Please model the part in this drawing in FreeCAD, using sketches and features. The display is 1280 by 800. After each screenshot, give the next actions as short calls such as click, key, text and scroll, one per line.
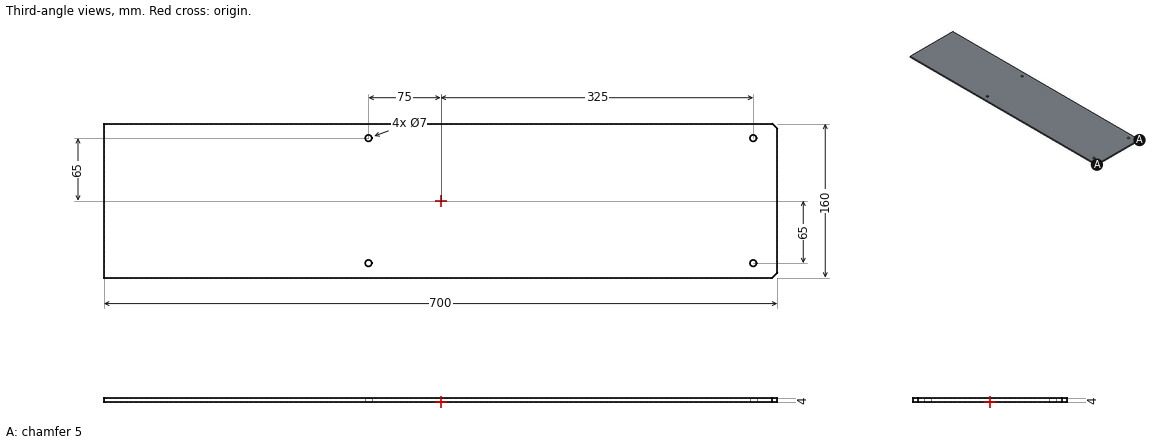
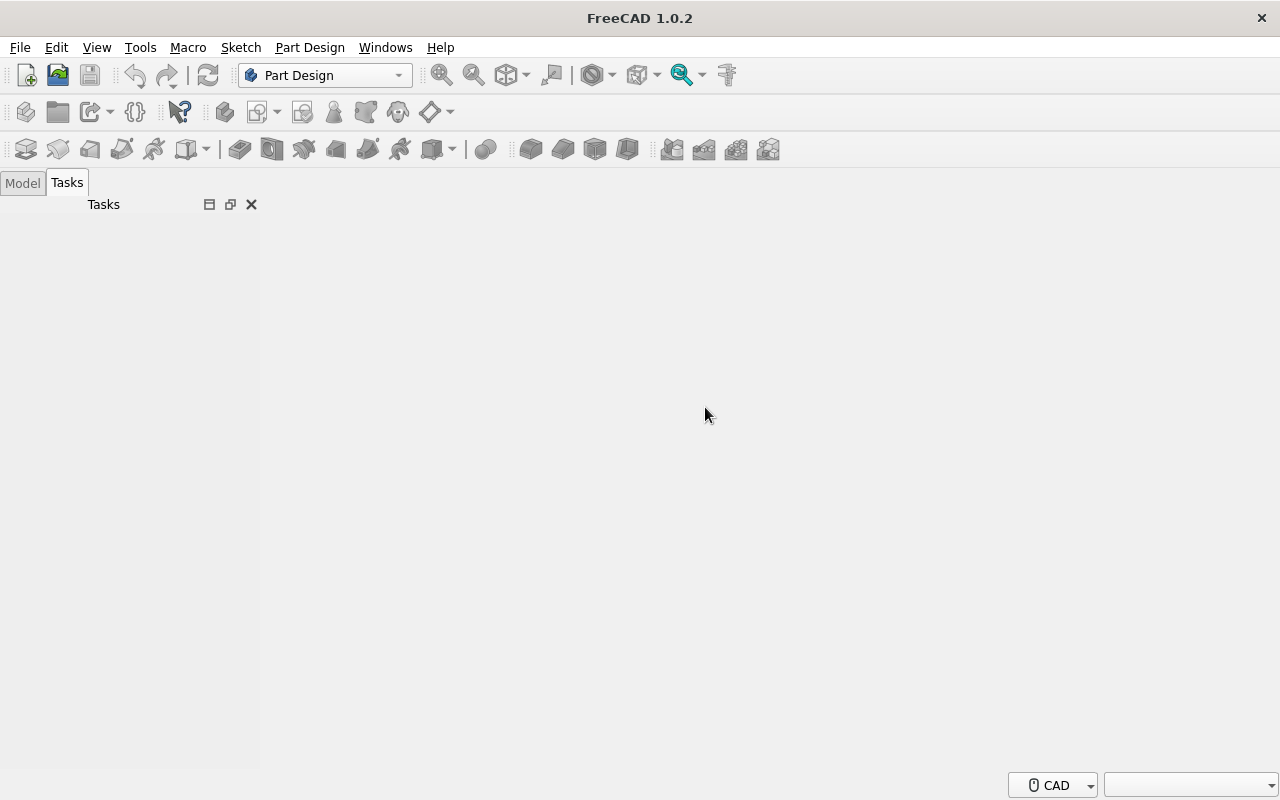
click(26, 76)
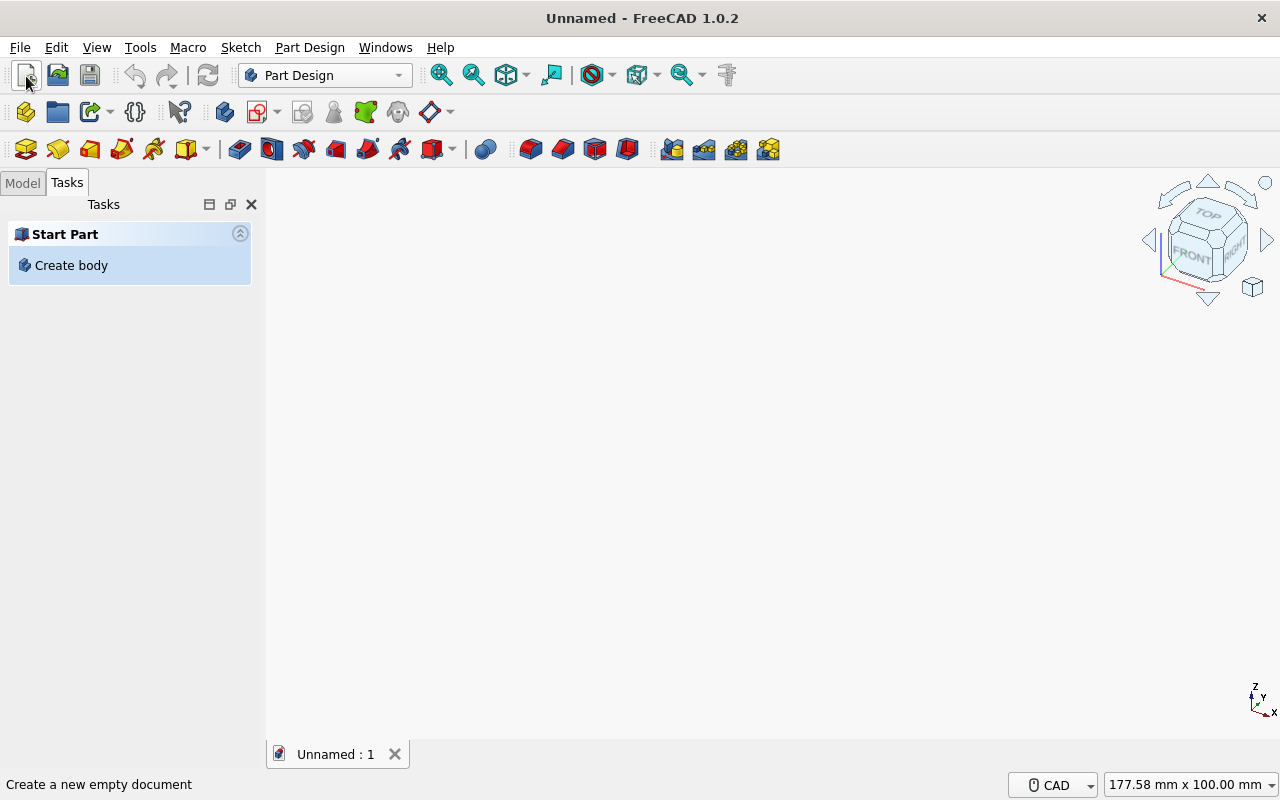
click(258, 112)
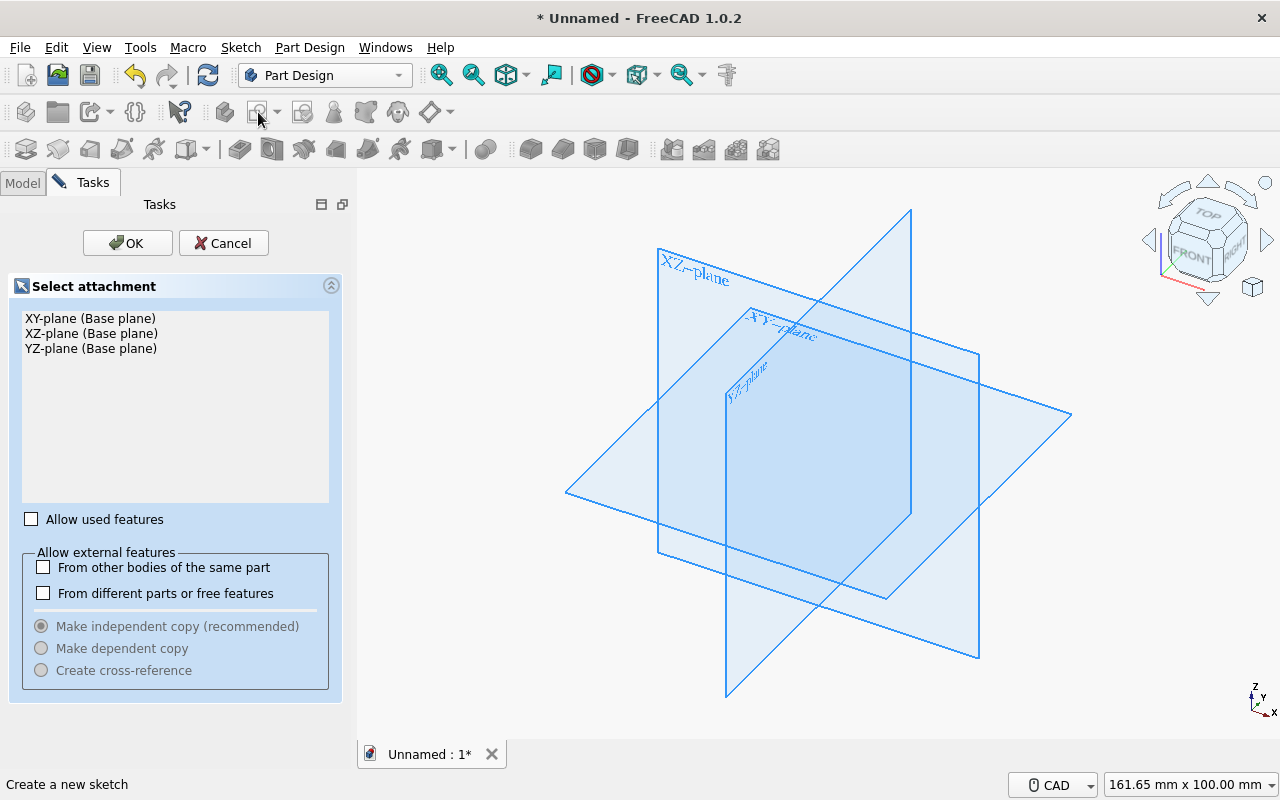
click(82, 318)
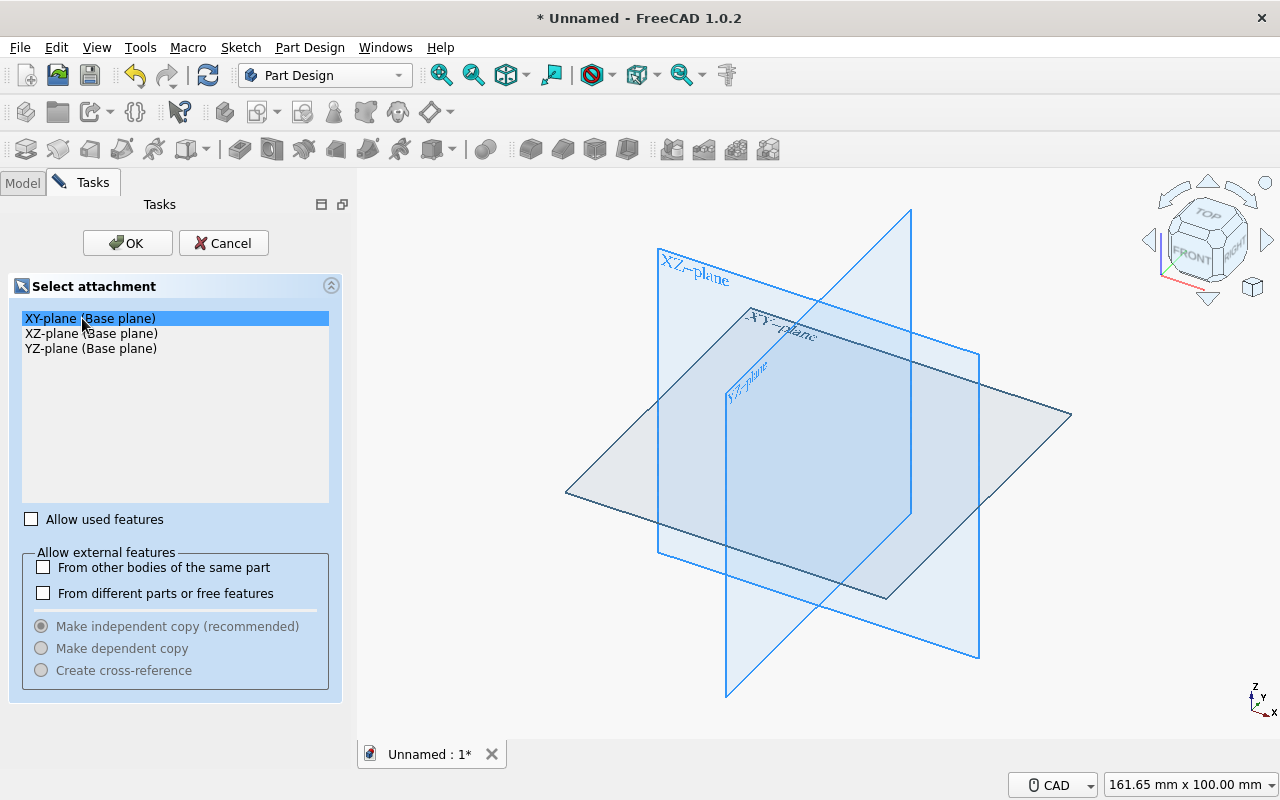
click(128, 243)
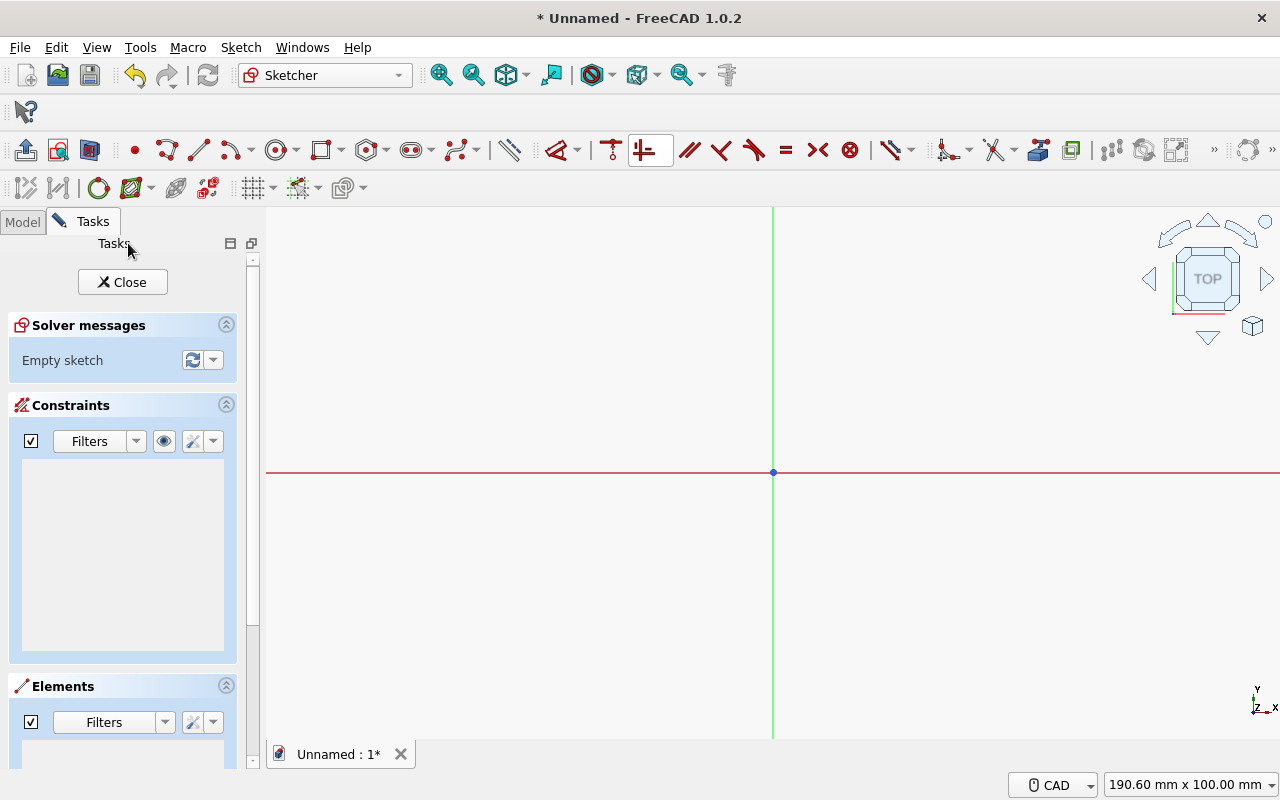
scroll(691, 473, down, 9)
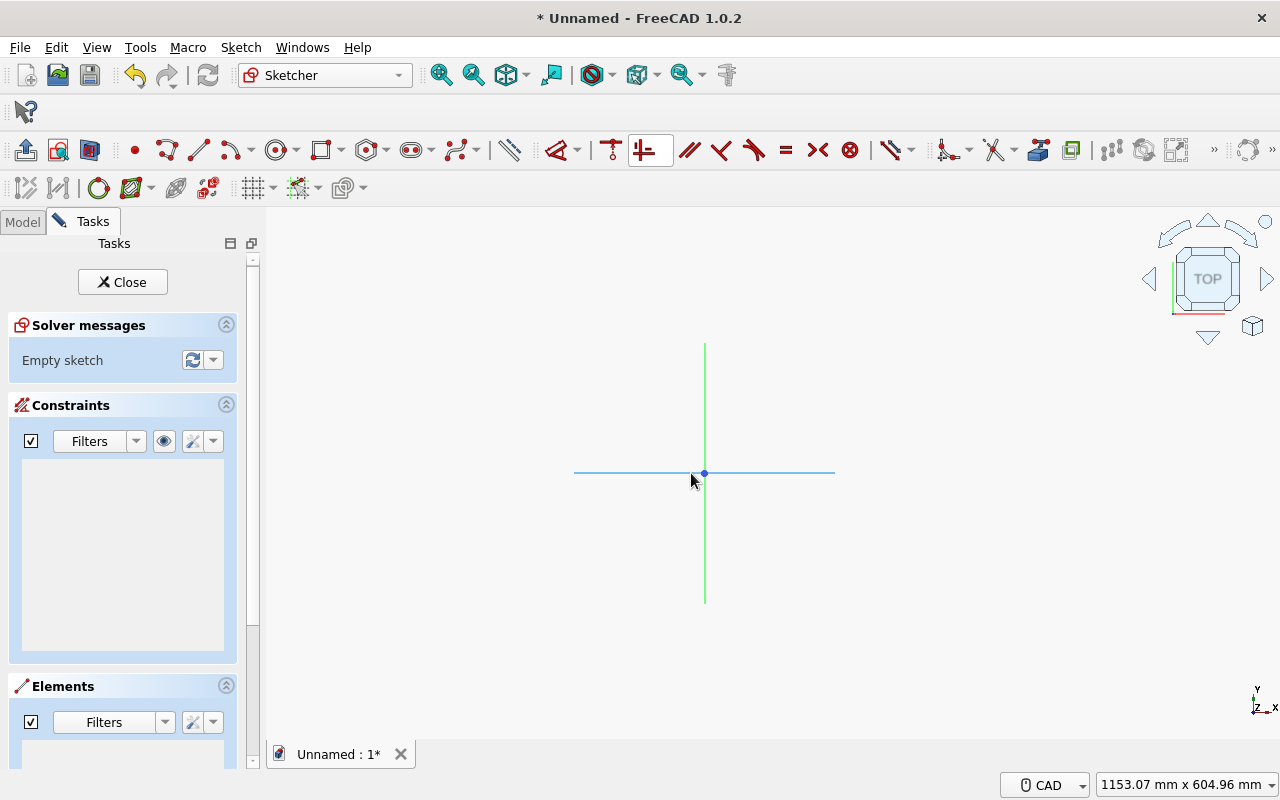
key(g)
key(v)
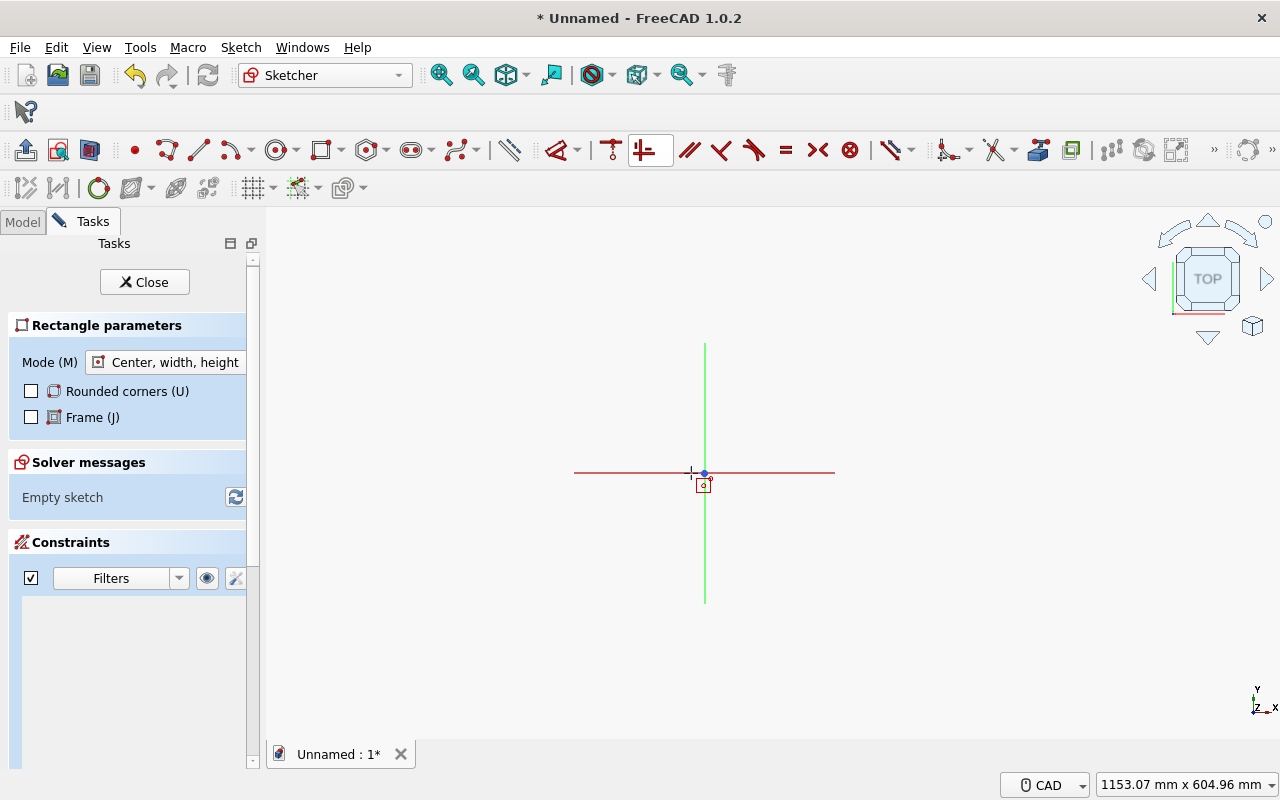
click(705, 473)
move(1013, 403)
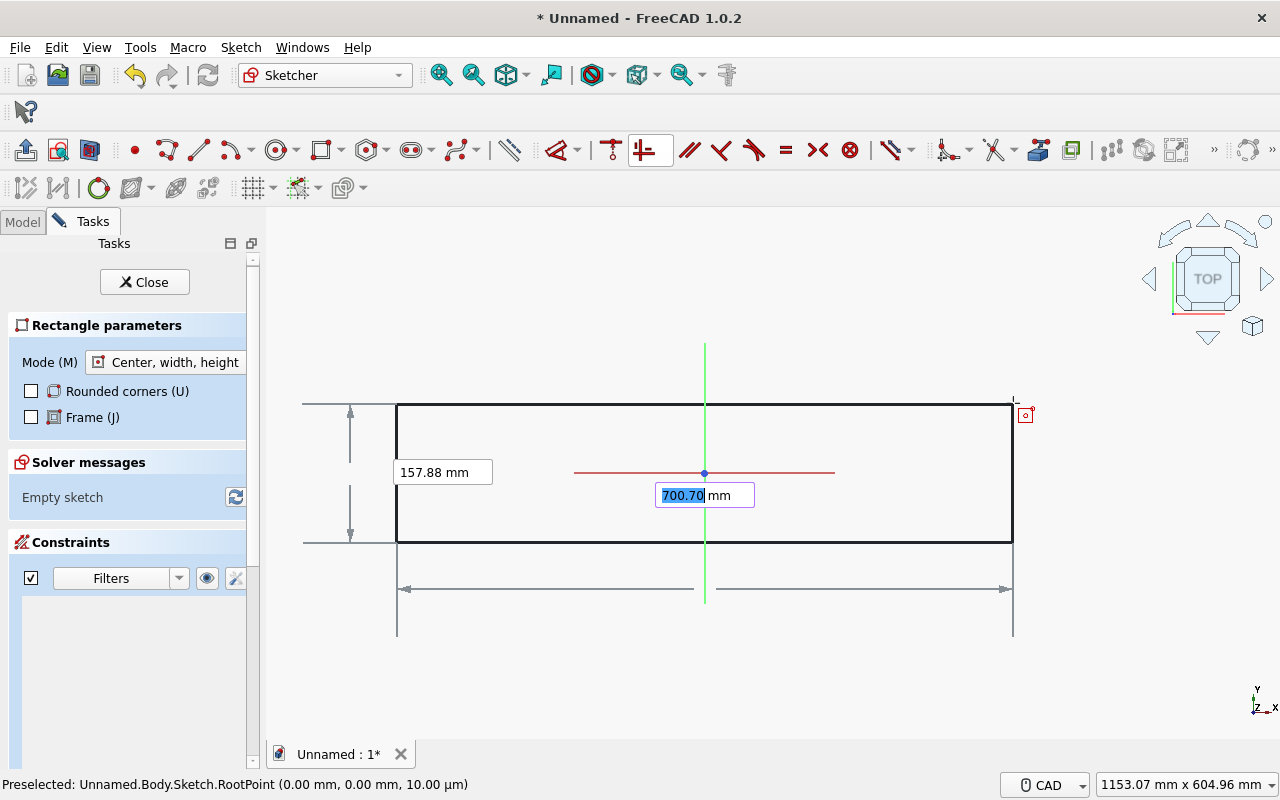
text(700)
key(Tab)
text(160)
key(Return)
key(Escape)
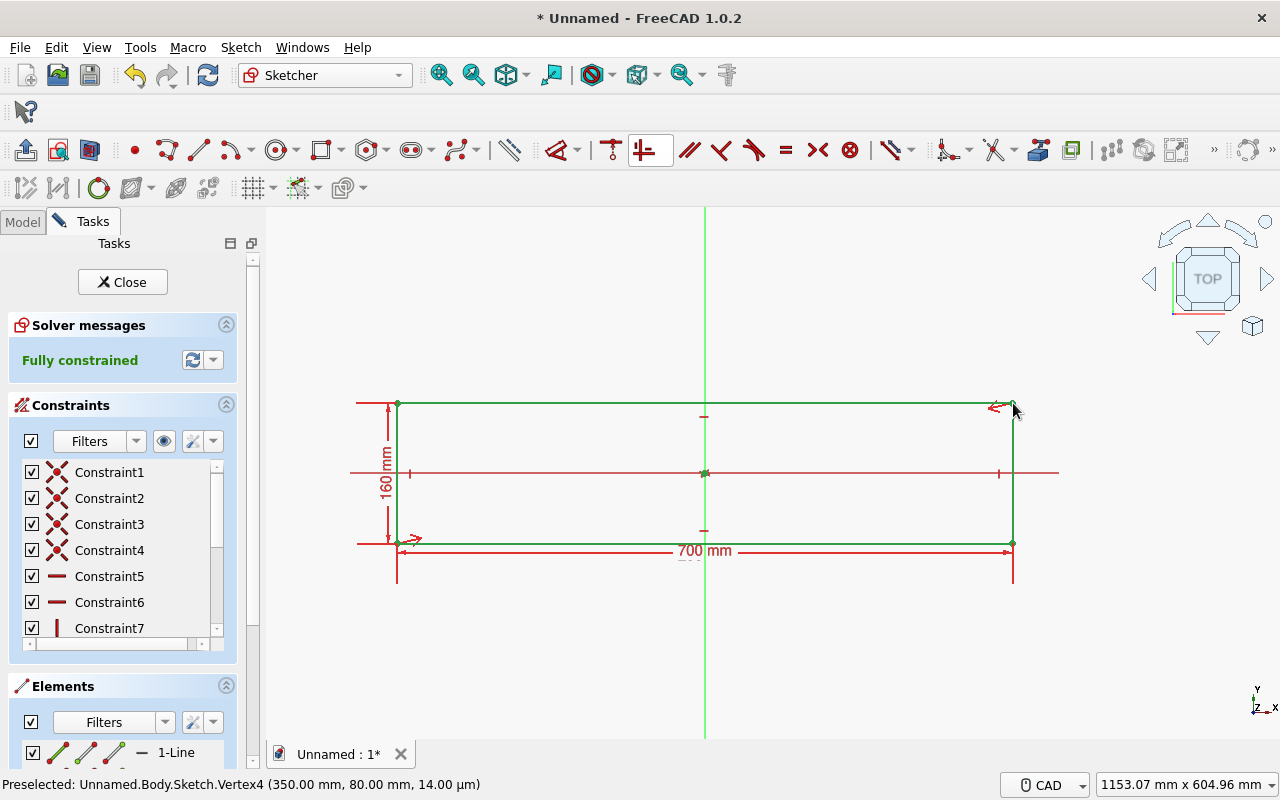
click(123, 282)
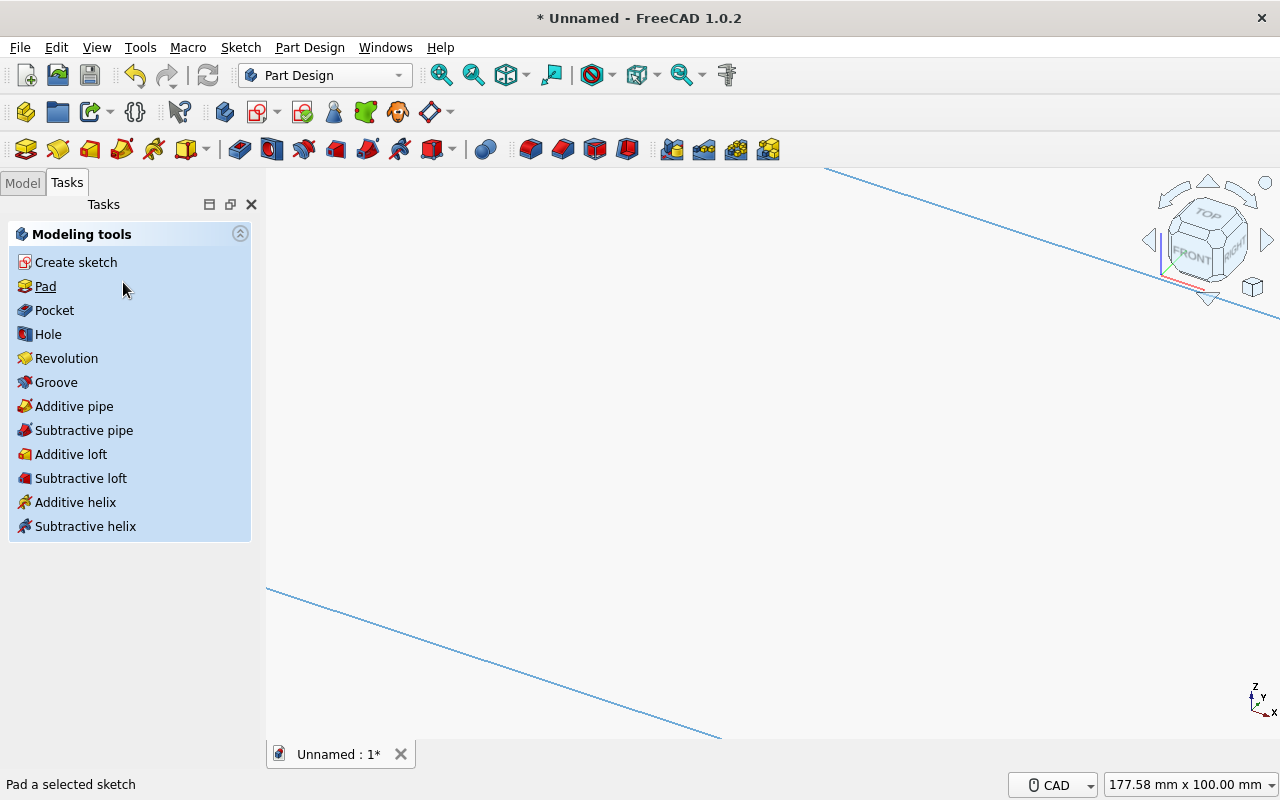
click(26, 150)